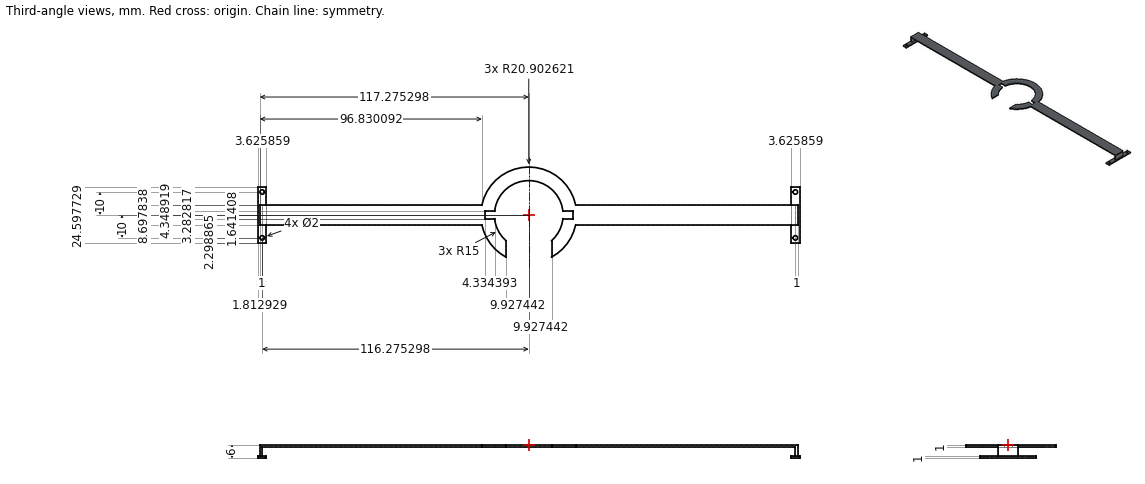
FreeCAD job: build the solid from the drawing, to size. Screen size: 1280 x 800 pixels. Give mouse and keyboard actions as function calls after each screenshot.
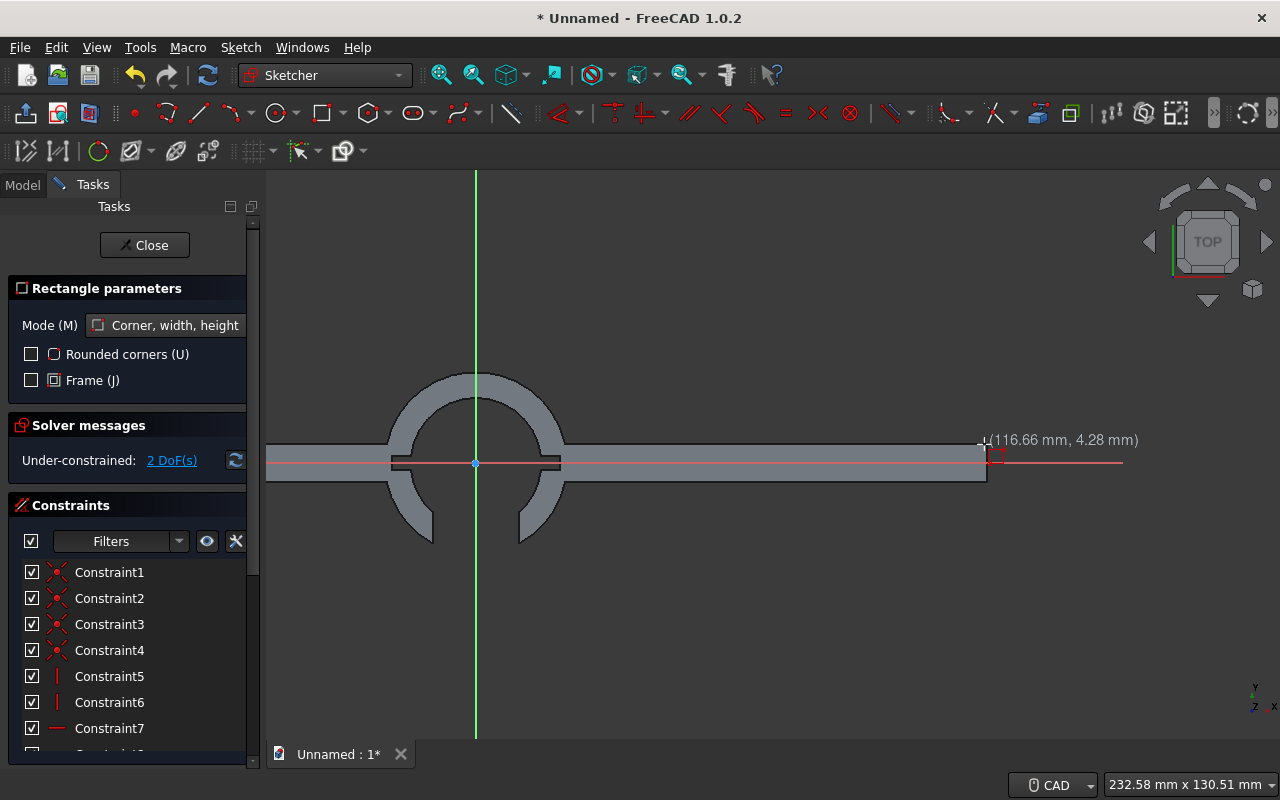
click(983, 444)
move(987, 482)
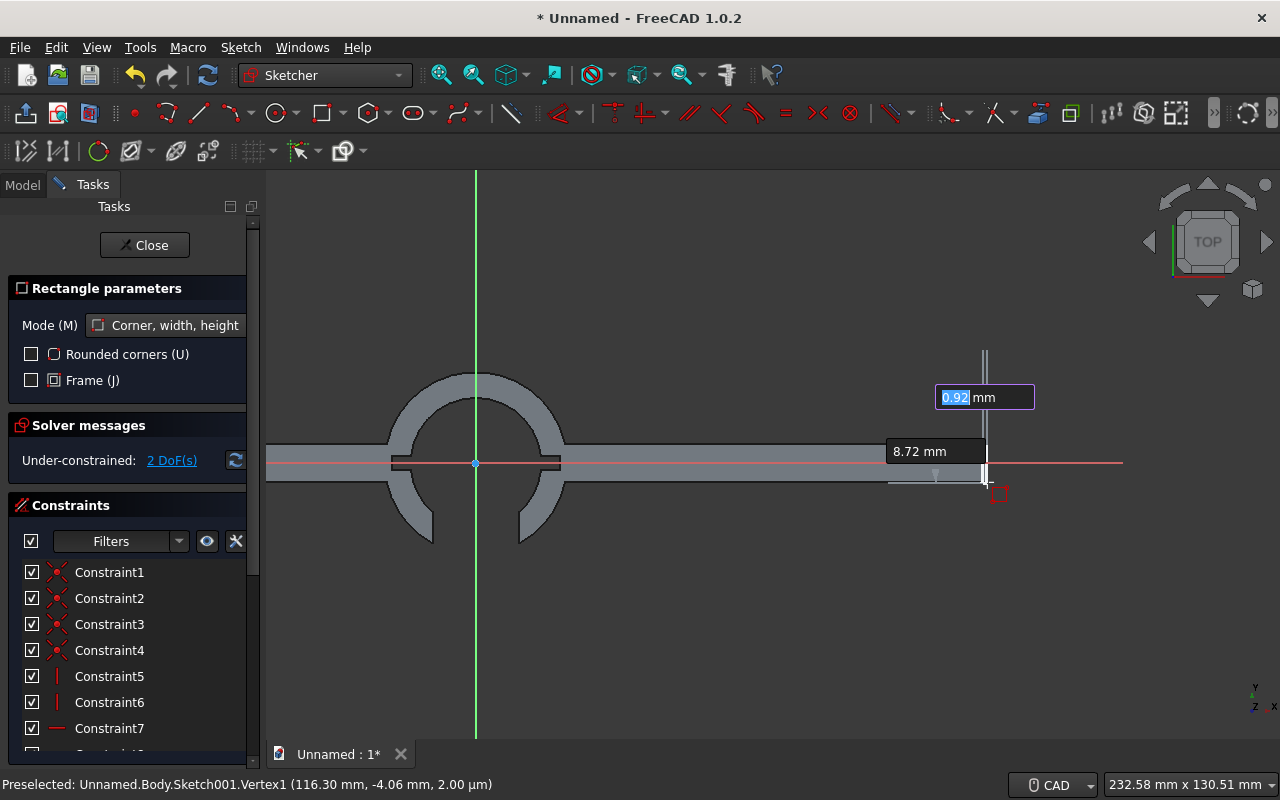
text(1)
key(Tab)
text(8.697838)
key(Return)
key(Escape)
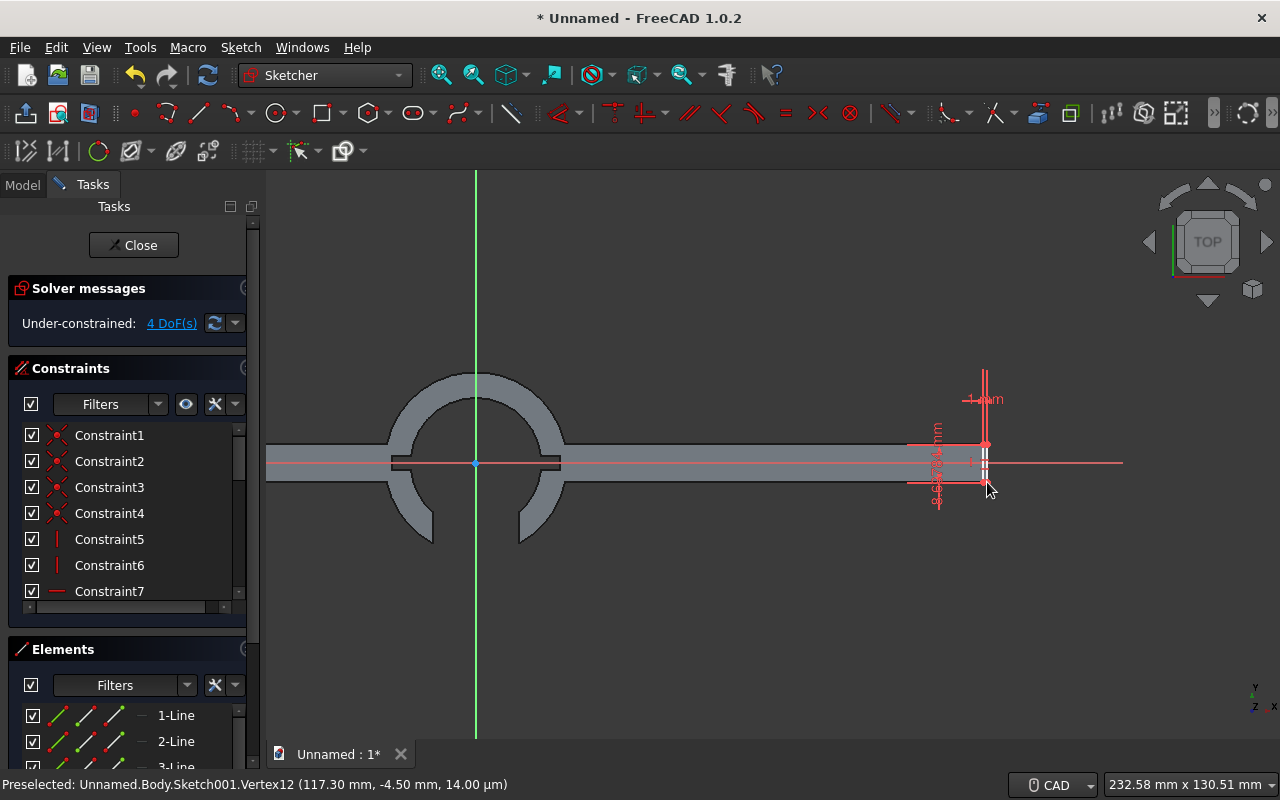
scroll(983, 444, down, 3)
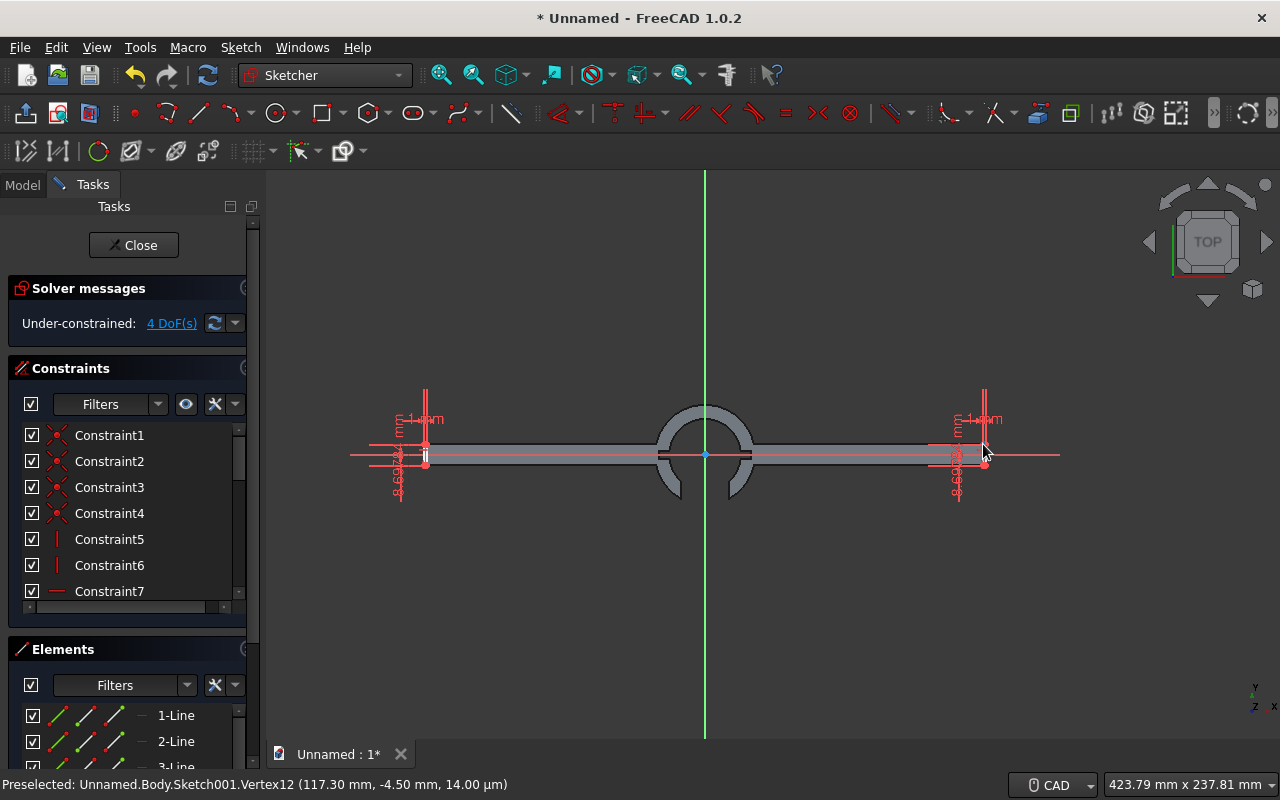
scroll(427, 445, up, 9)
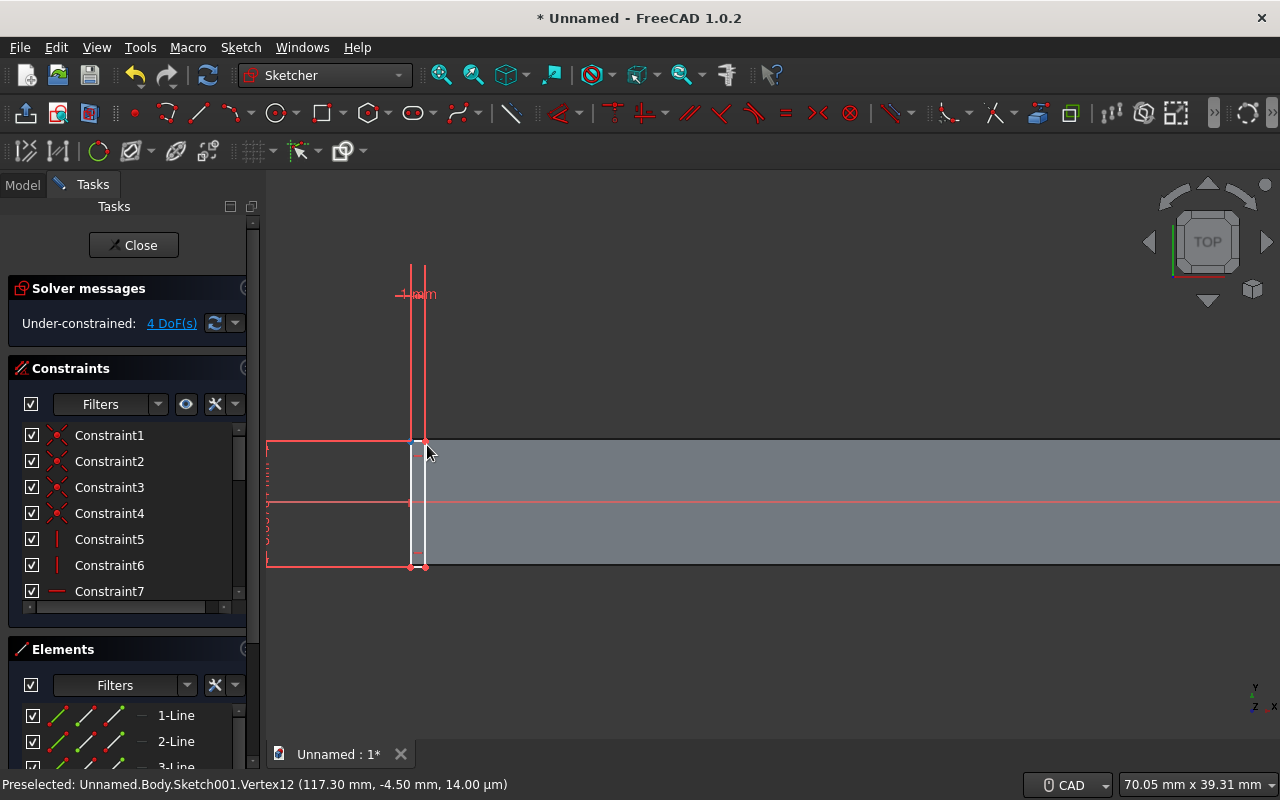
click(425, 441)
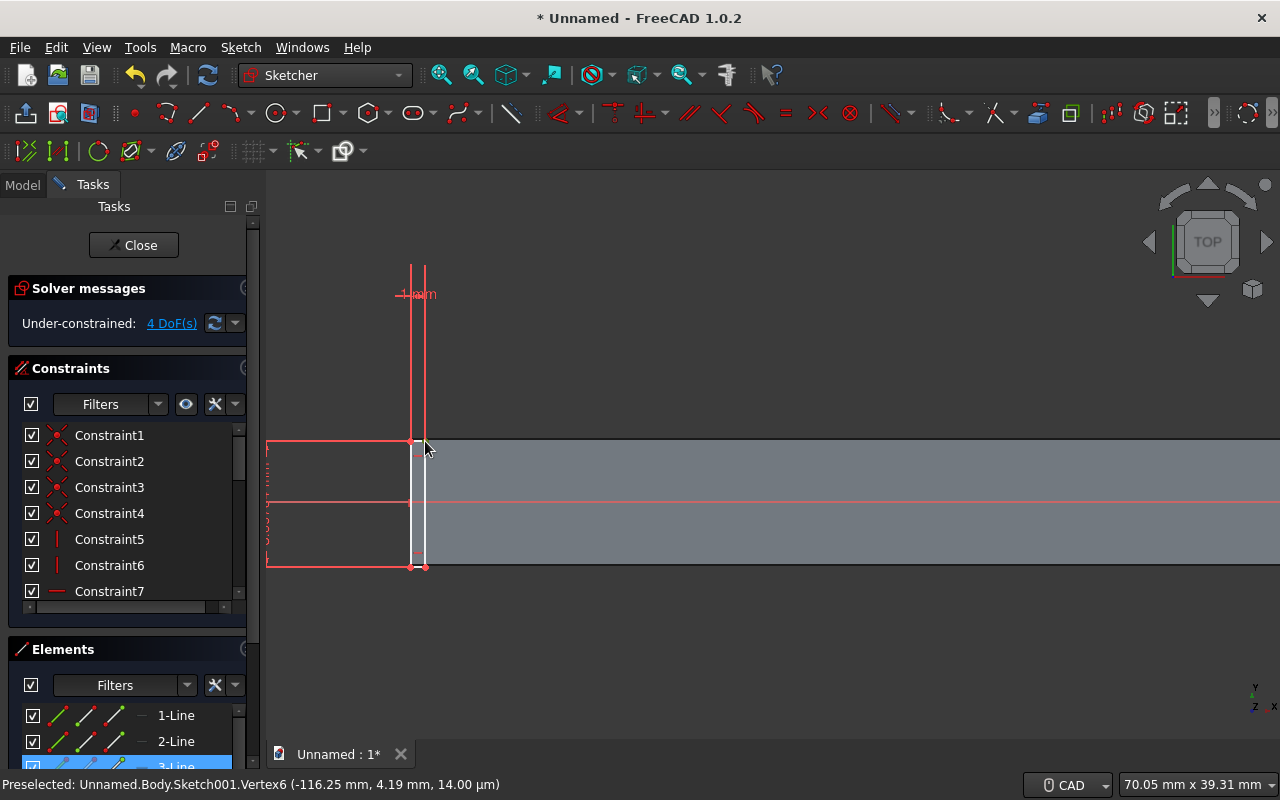
scroll(427, 445, down, 9)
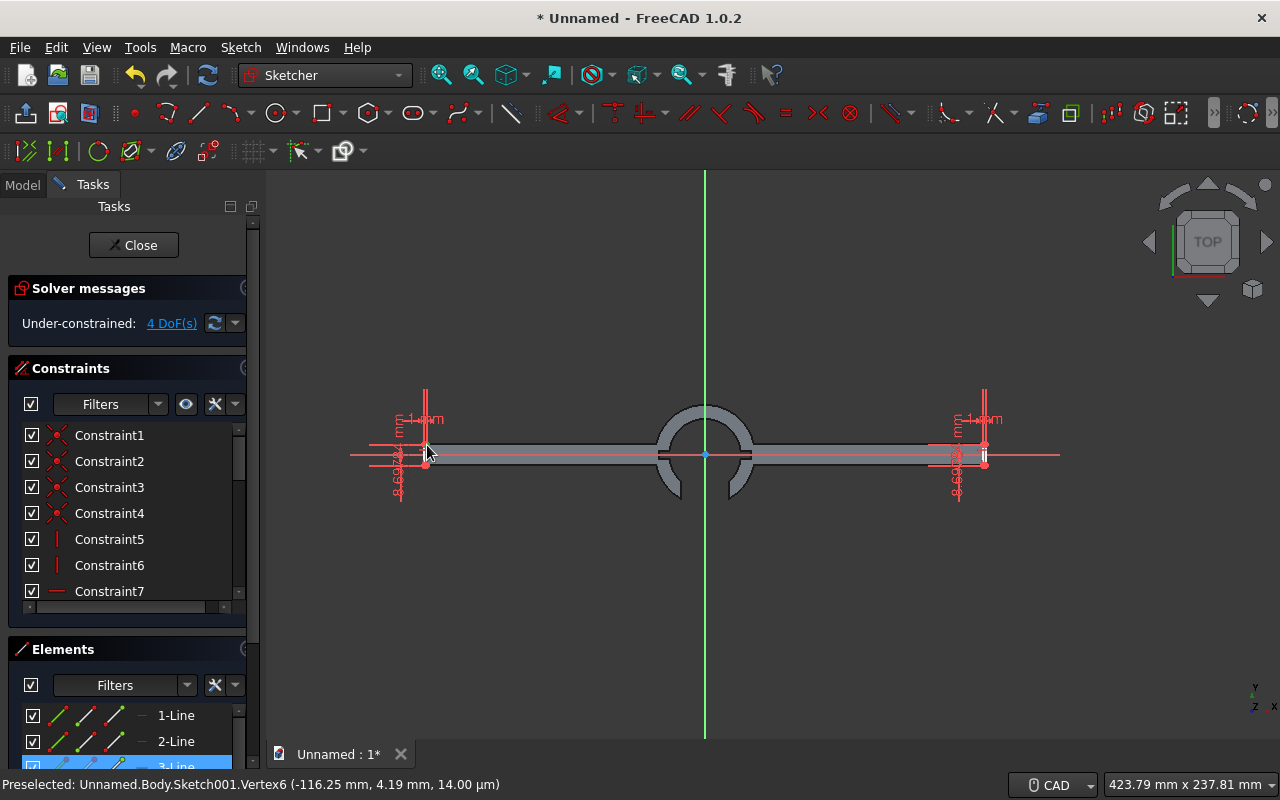
scroll(983, 445, up, 9)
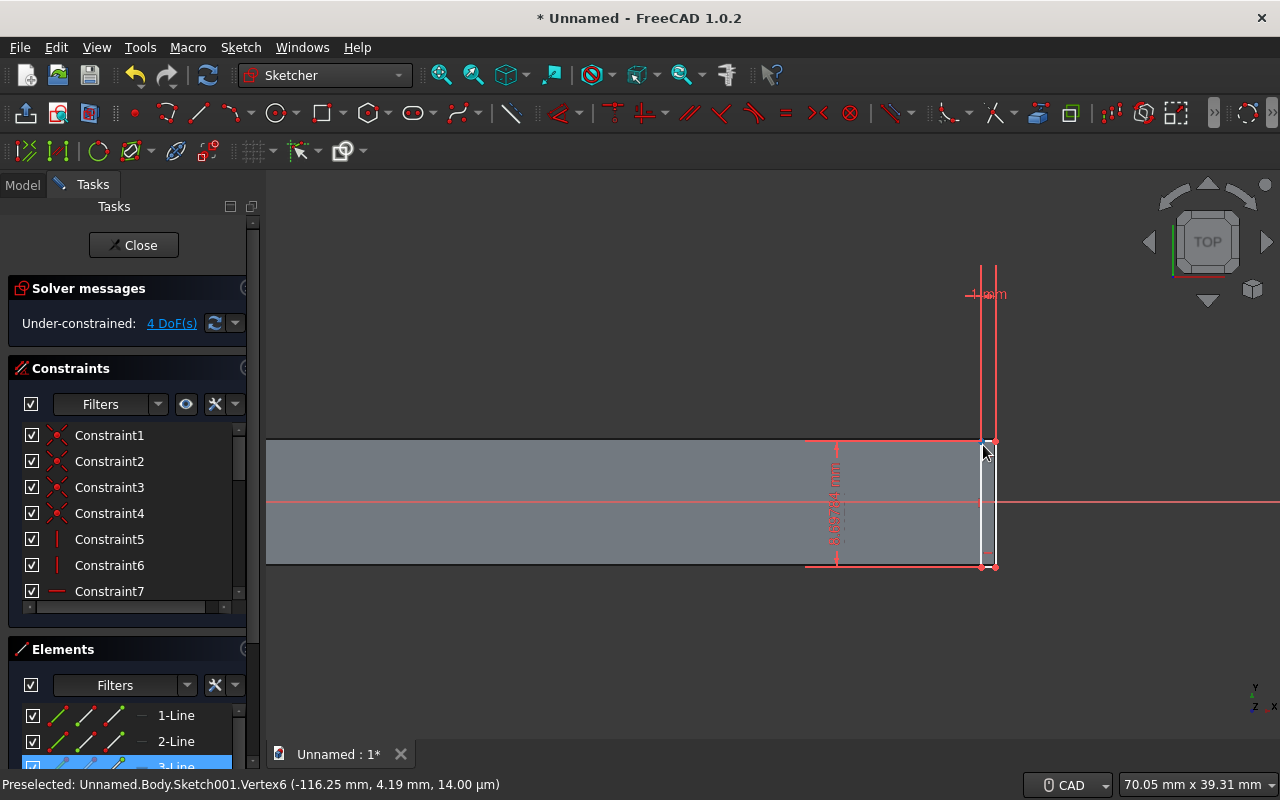
click(981, 441)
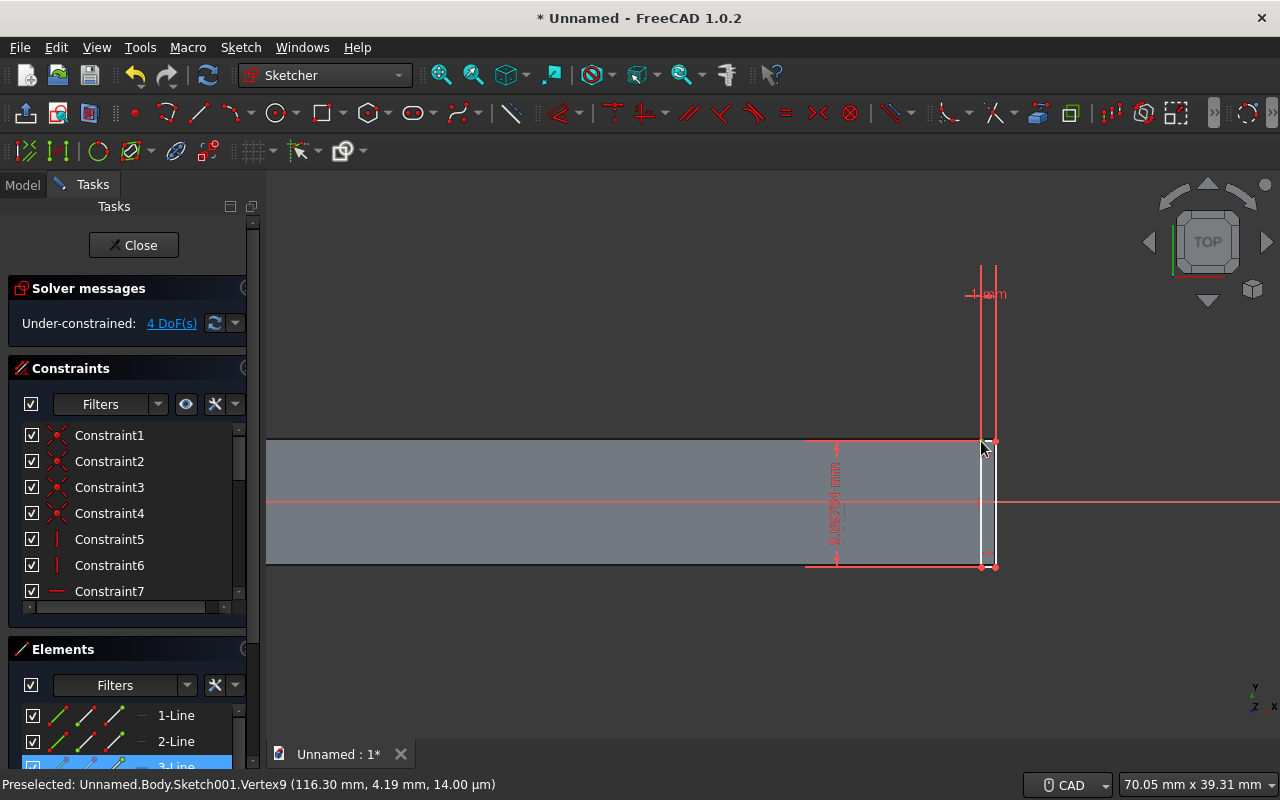
scroll(983, 445, down, 9)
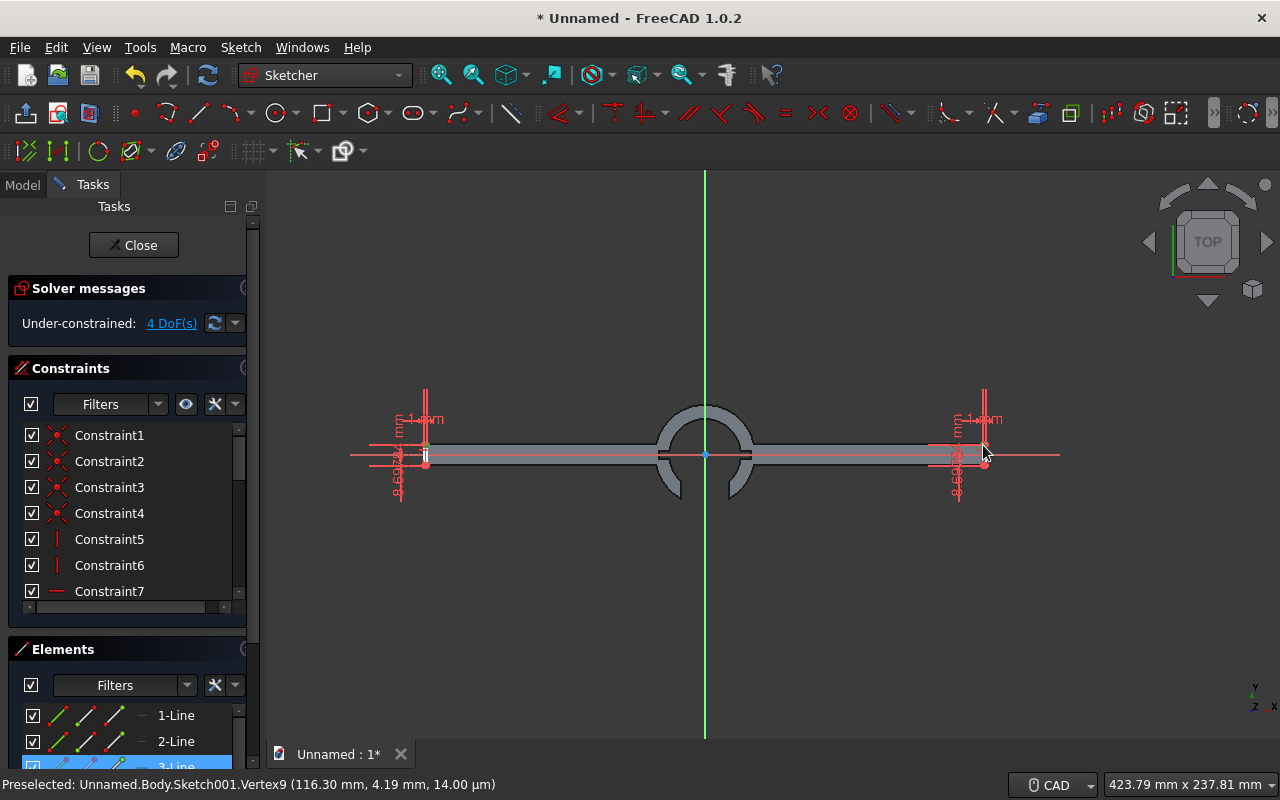
click(705, 674)